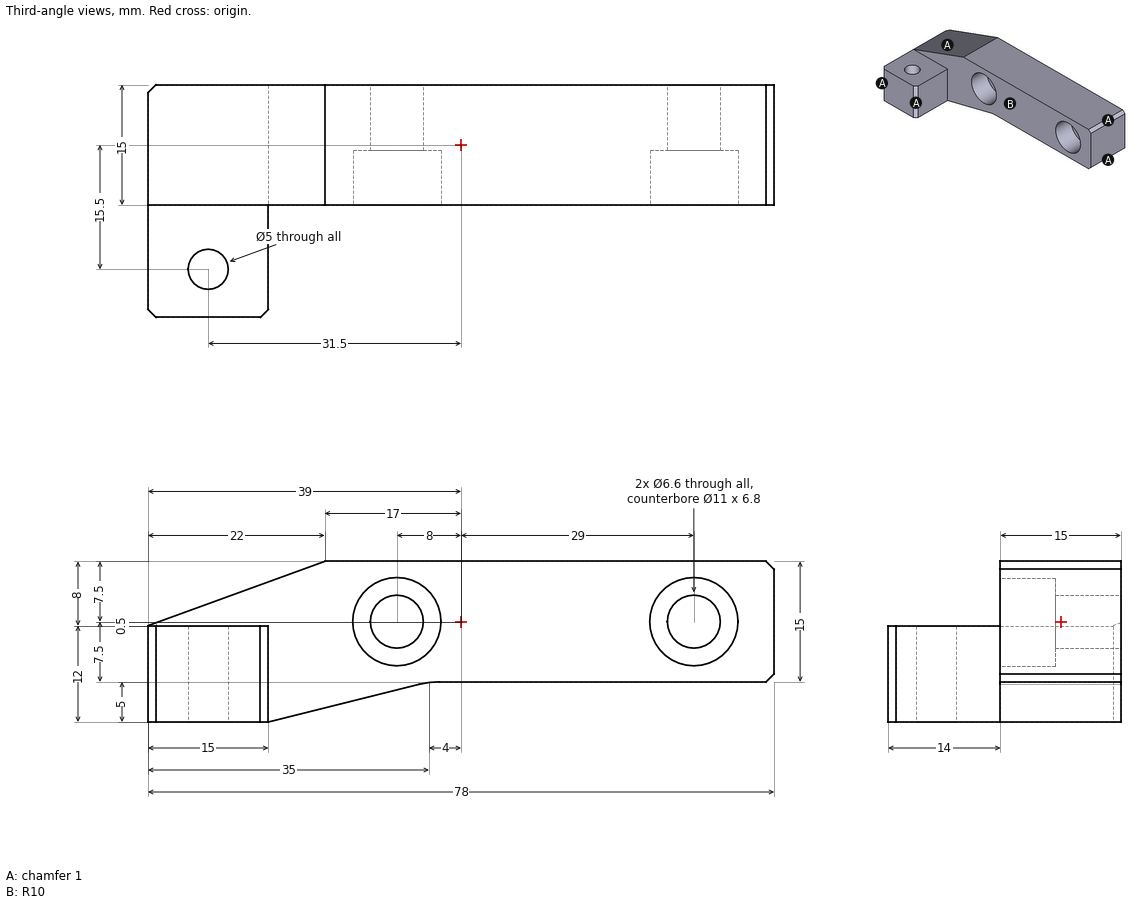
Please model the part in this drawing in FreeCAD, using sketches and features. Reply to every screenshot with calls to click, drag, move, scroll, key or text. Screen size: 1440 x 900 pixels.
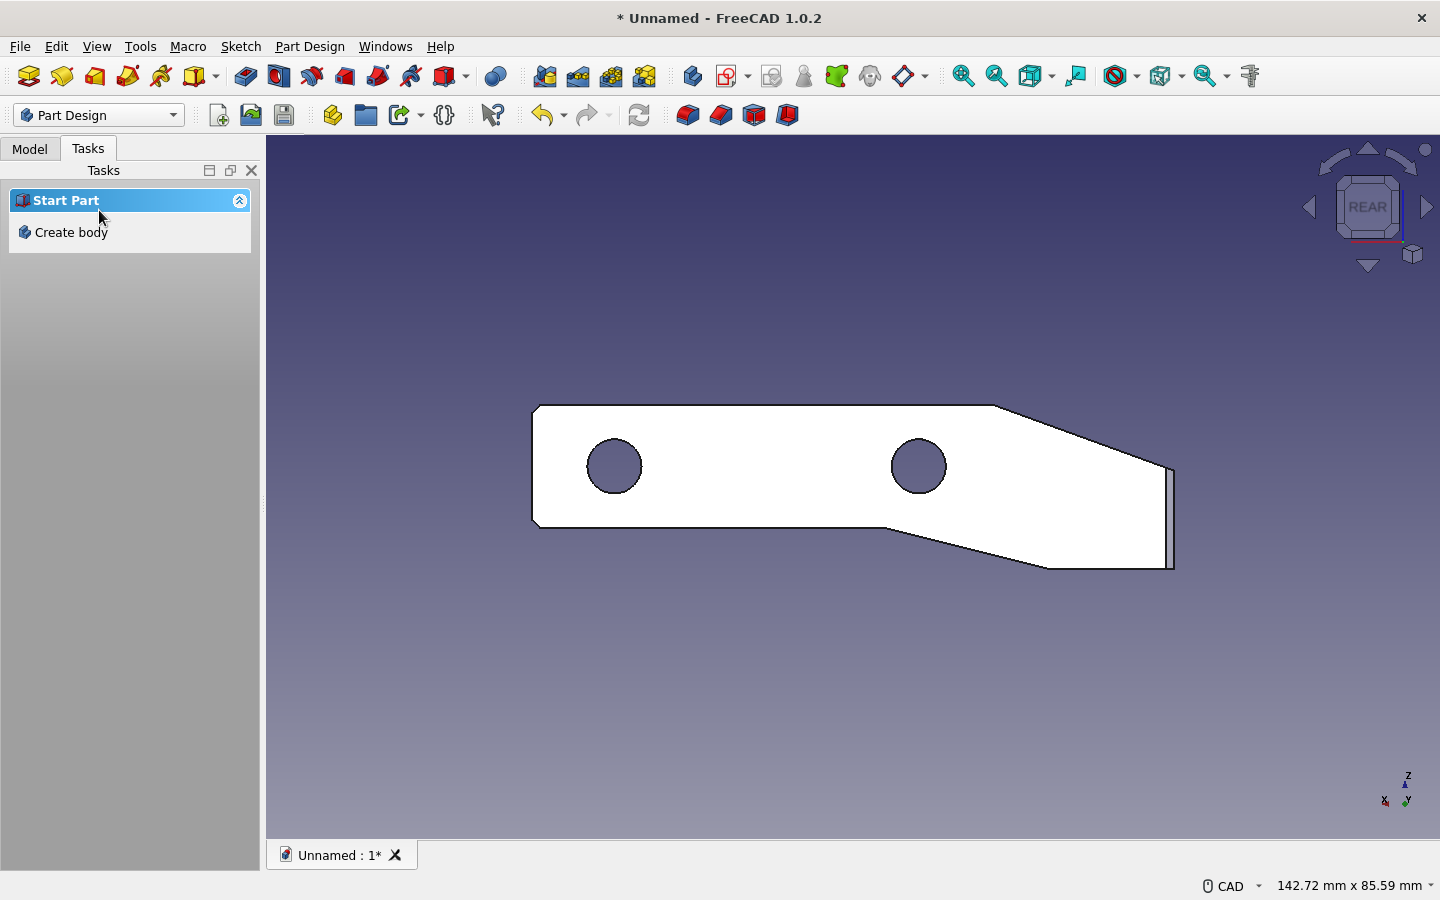
key(6)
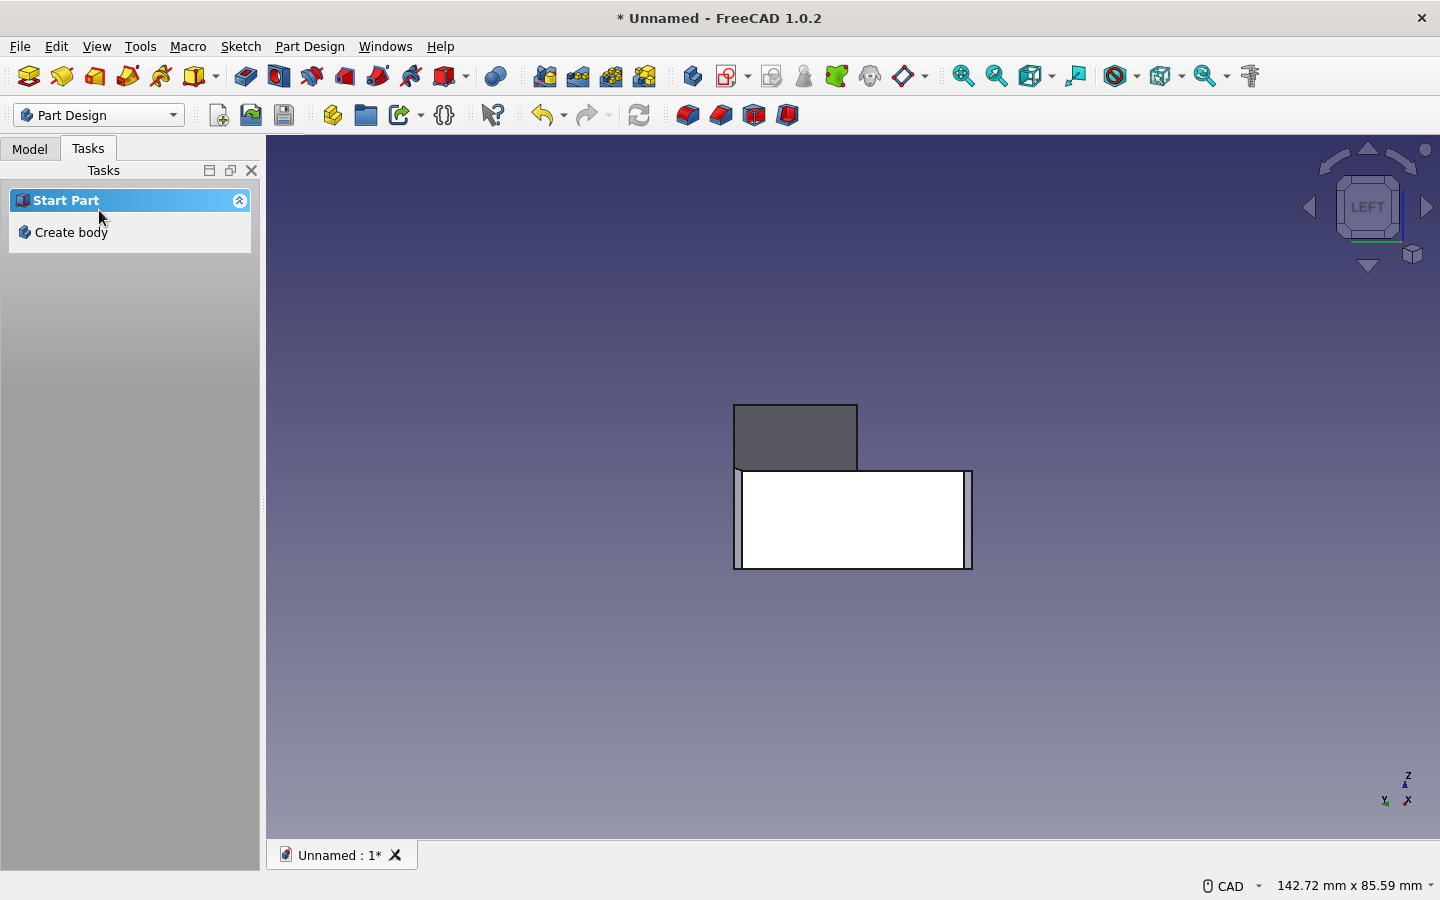
click(964, 76)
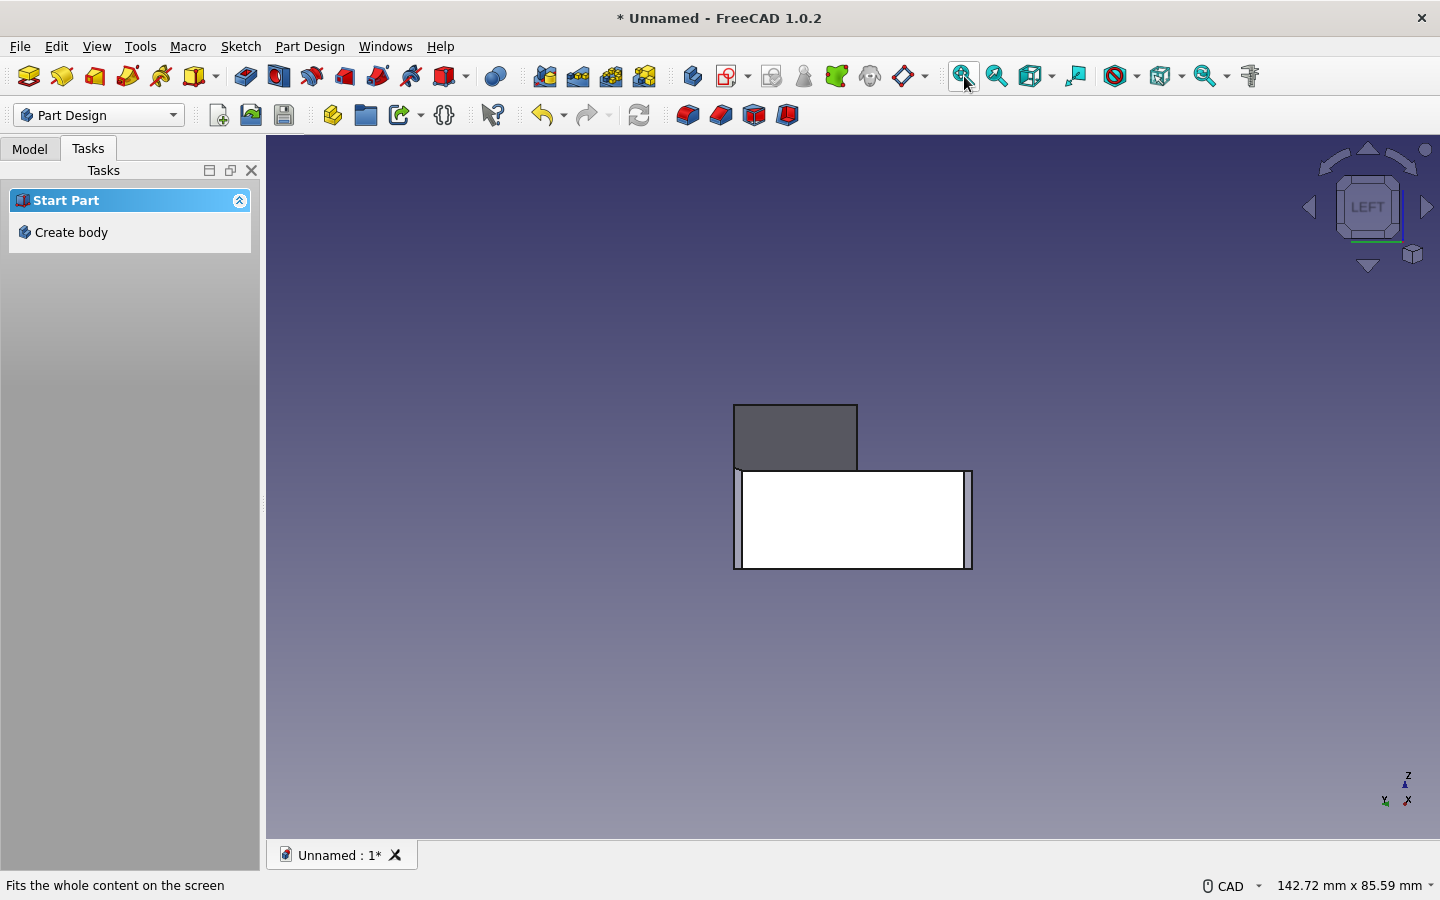
key(v)
key(3)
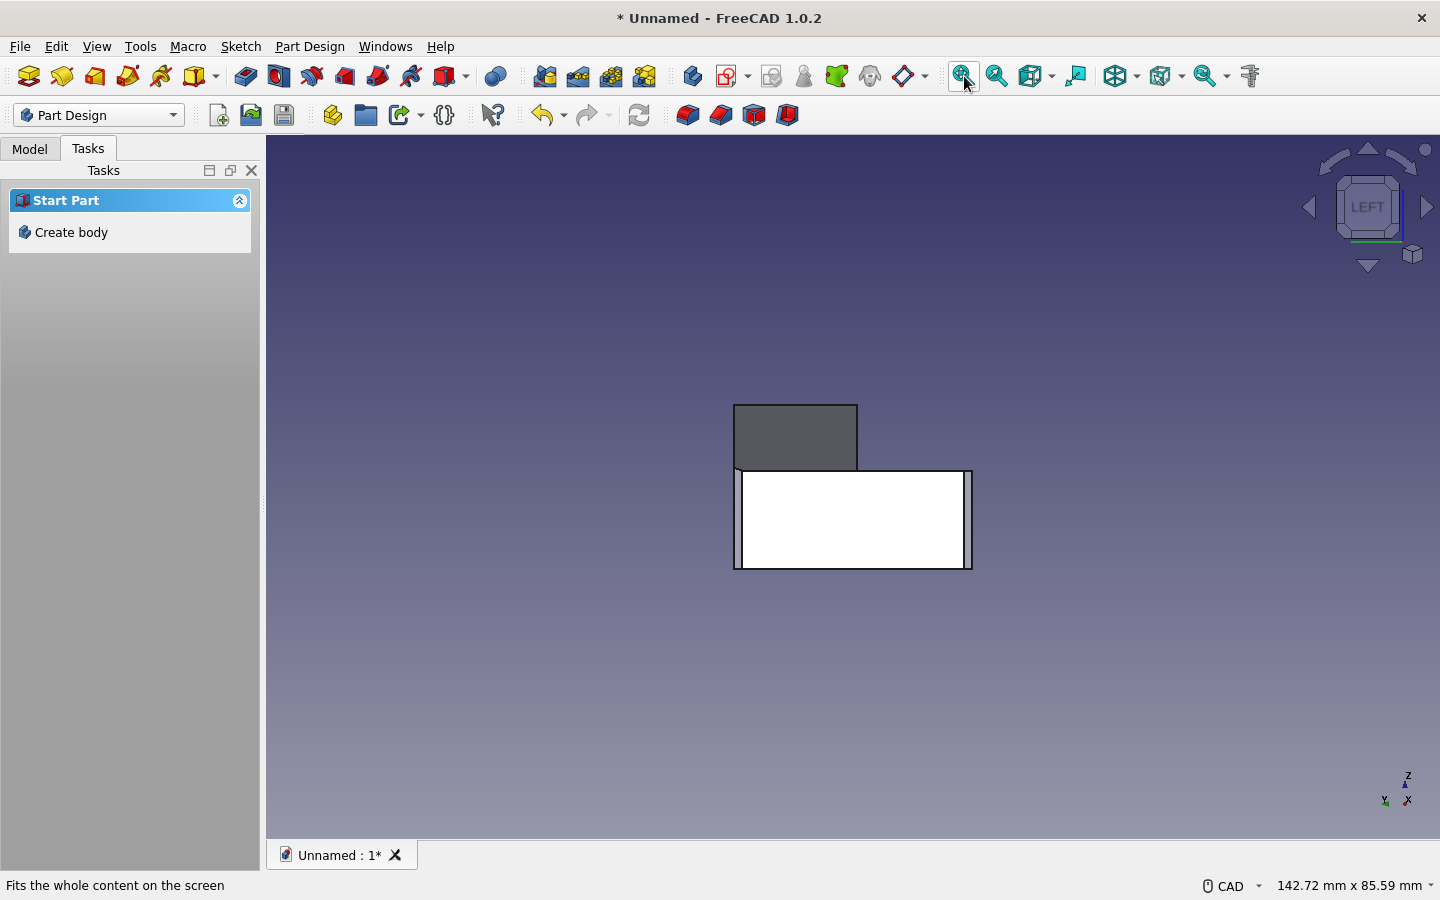
key(0)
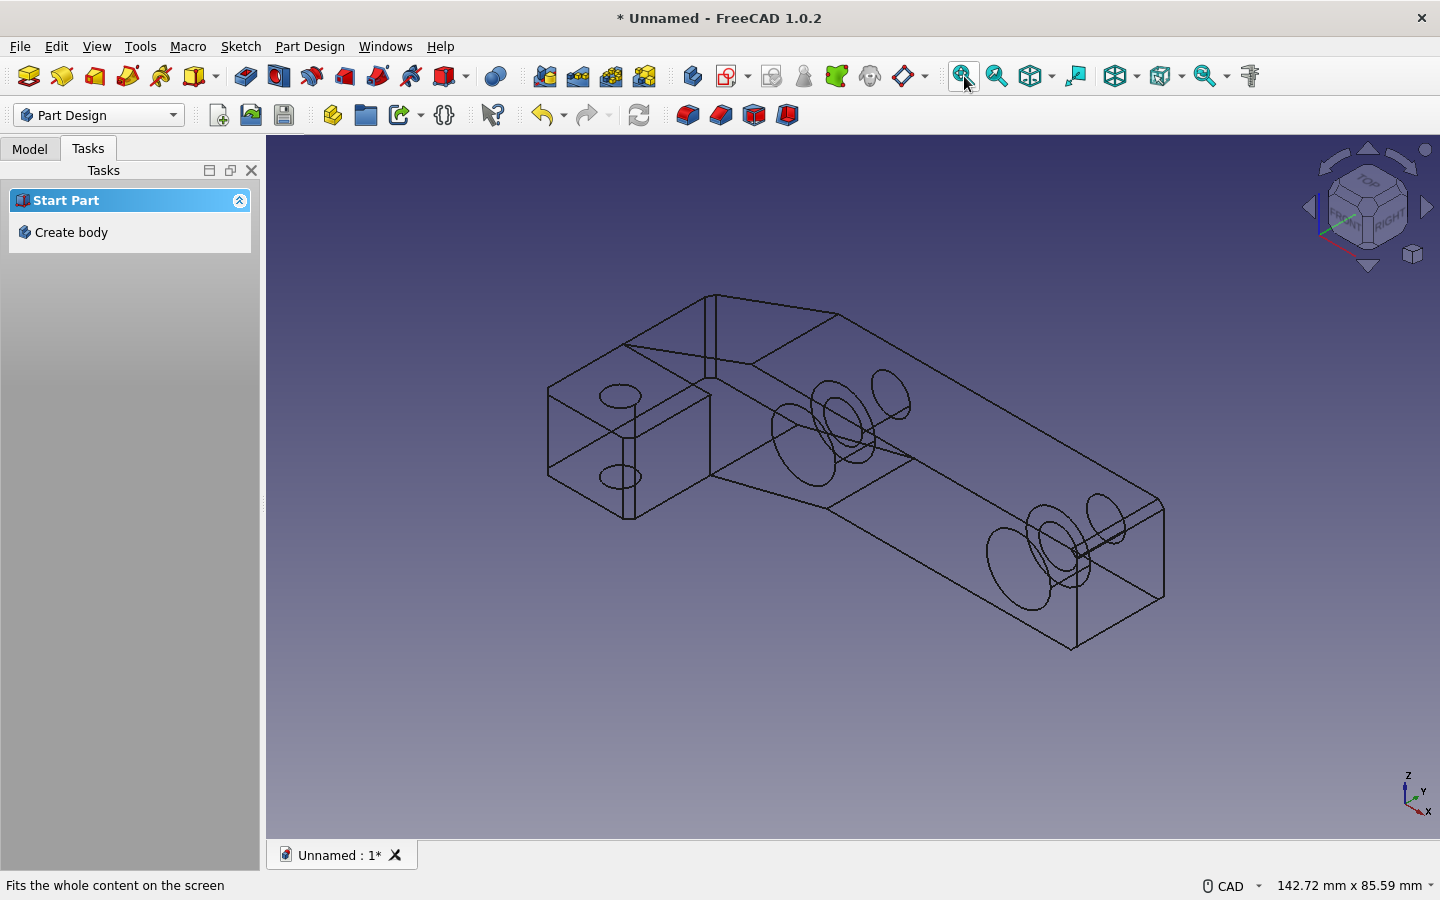
click(870, 483)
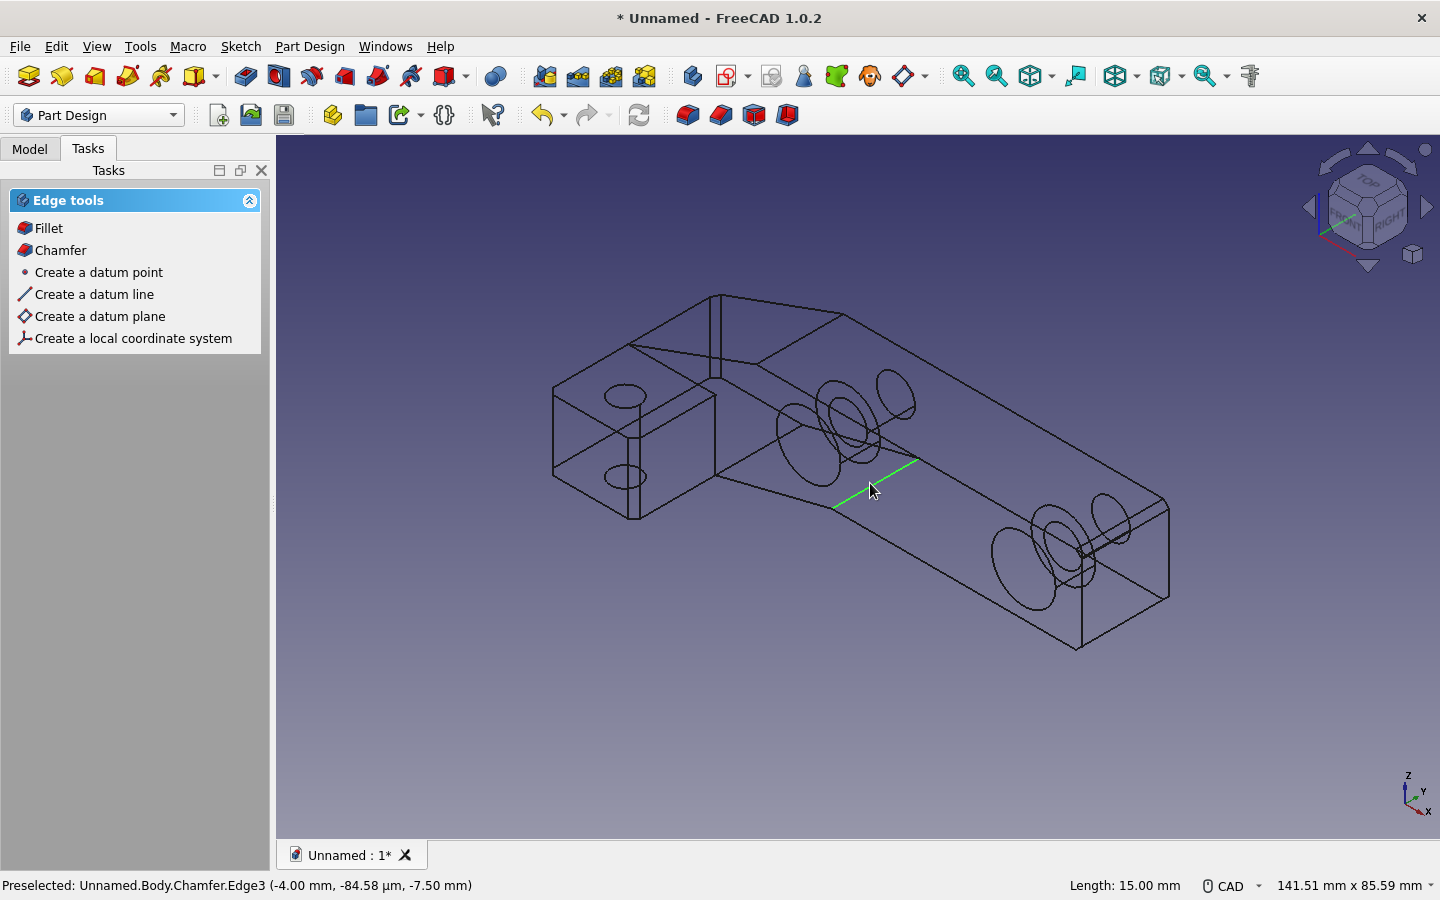
key(v)
key(1)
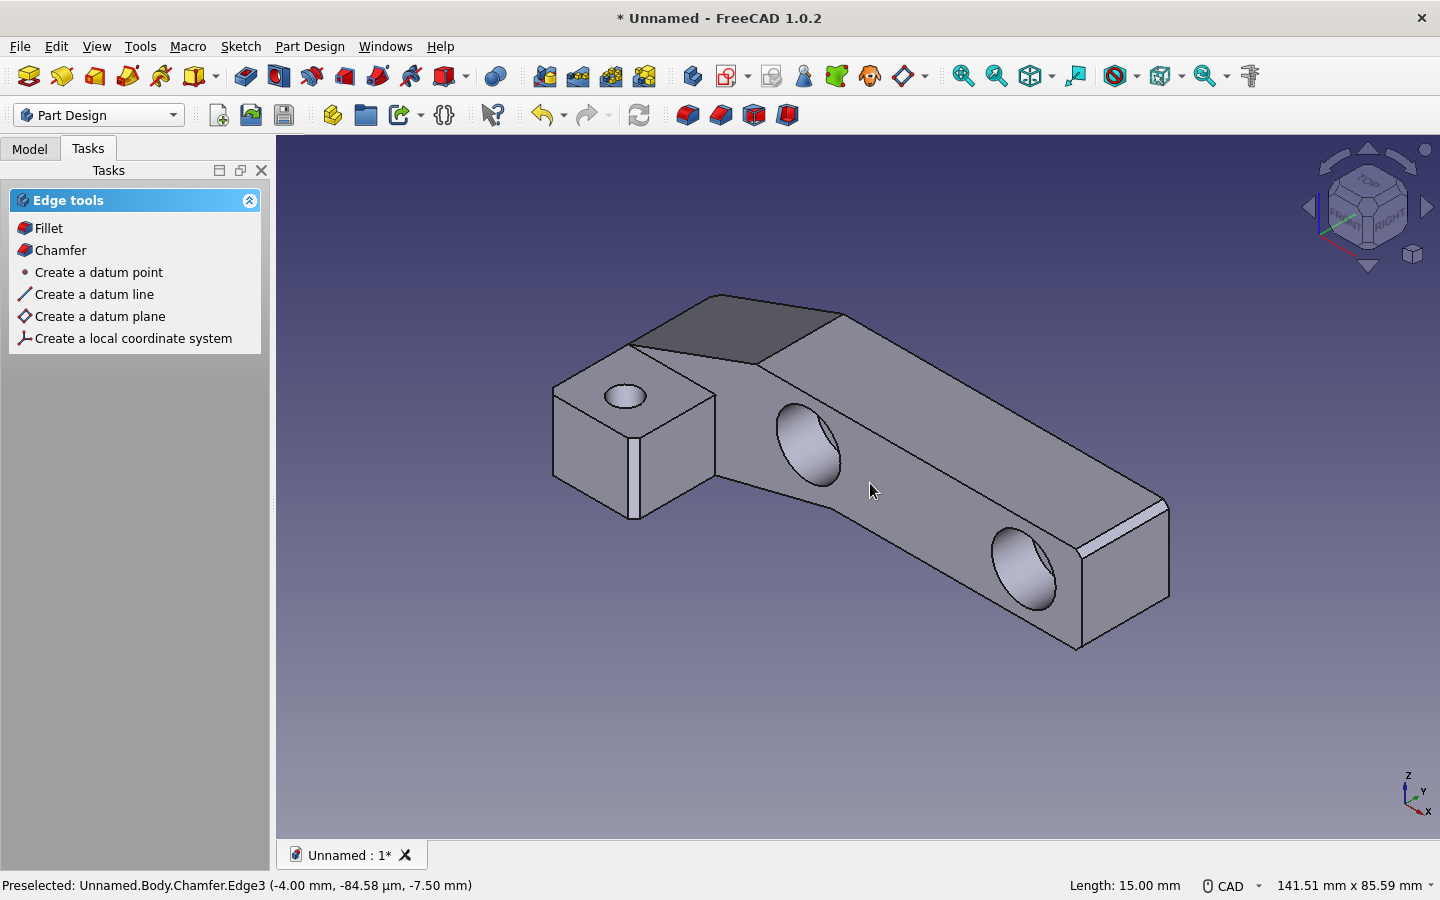
click(688, 116)